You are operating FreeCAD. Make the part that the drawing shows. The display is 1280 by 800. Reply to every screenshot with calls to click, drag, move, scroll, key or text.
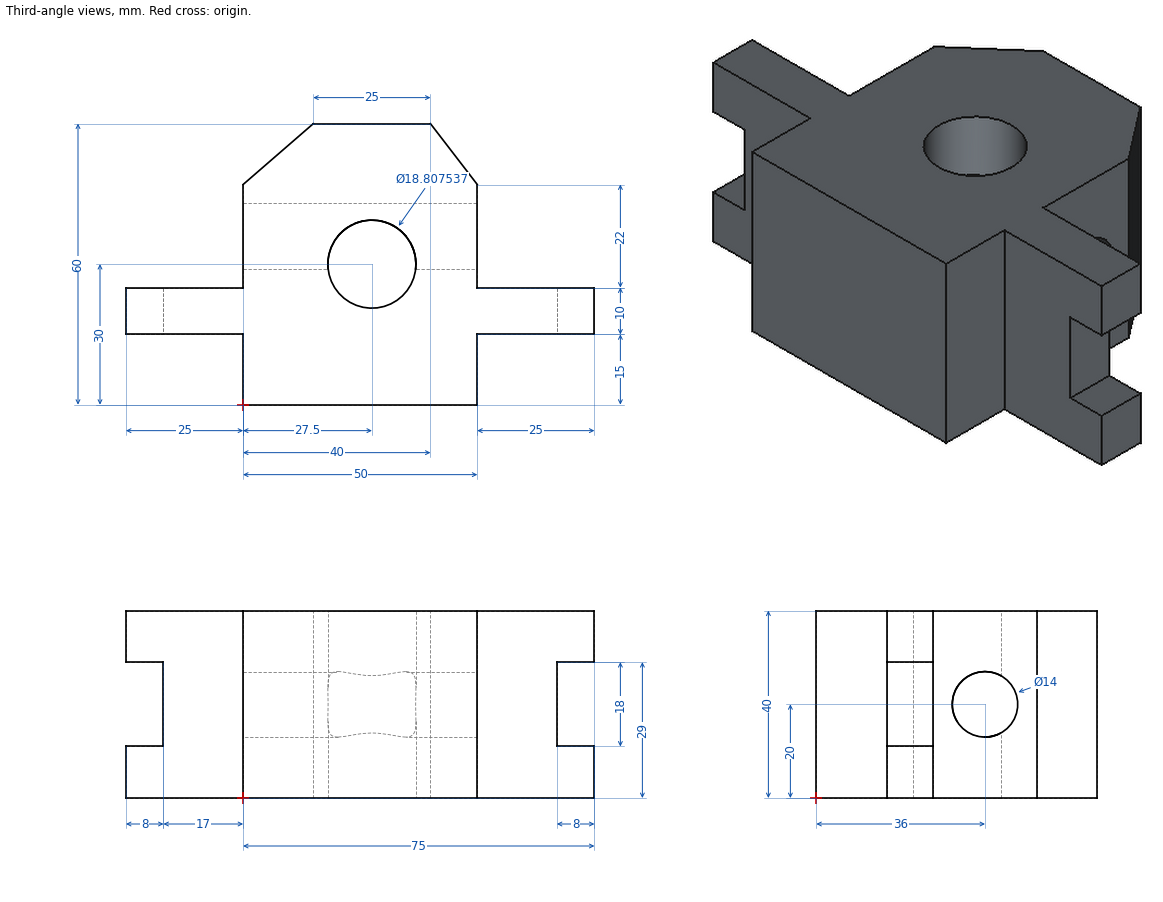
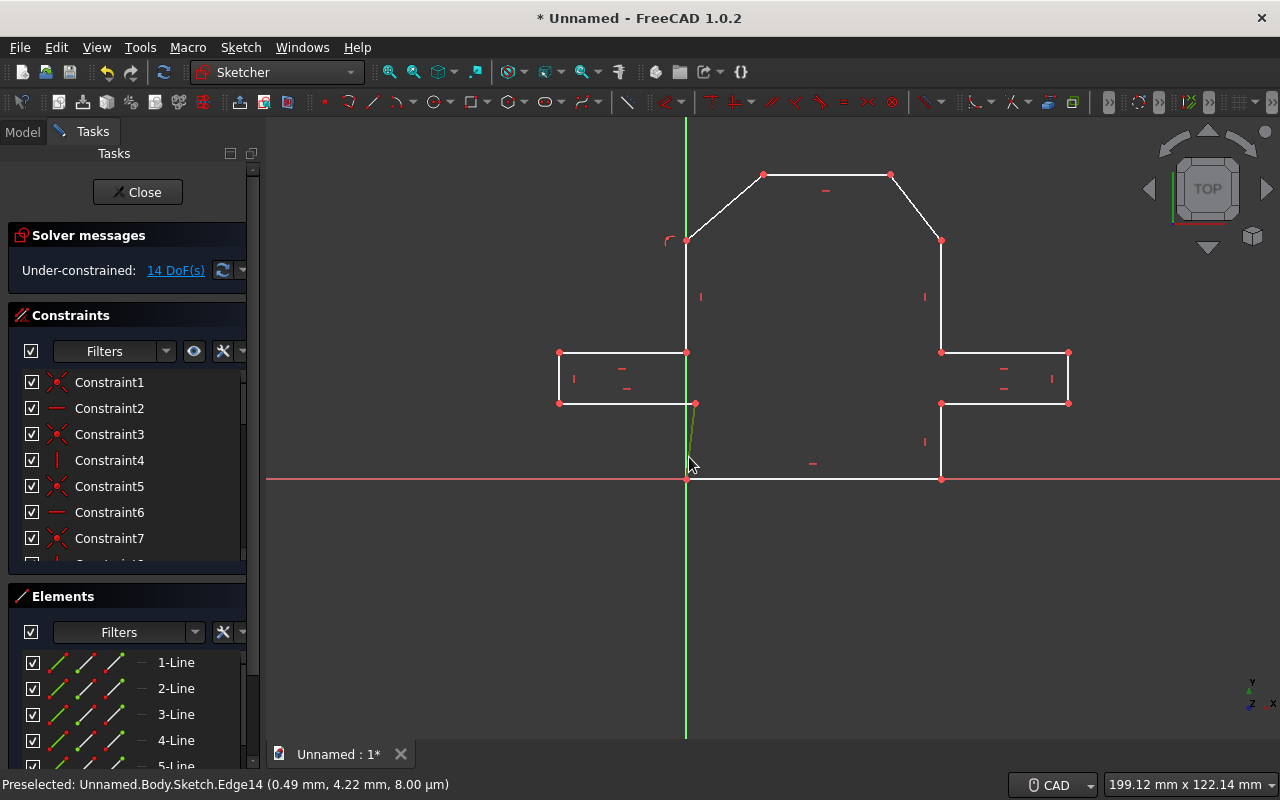
key(v)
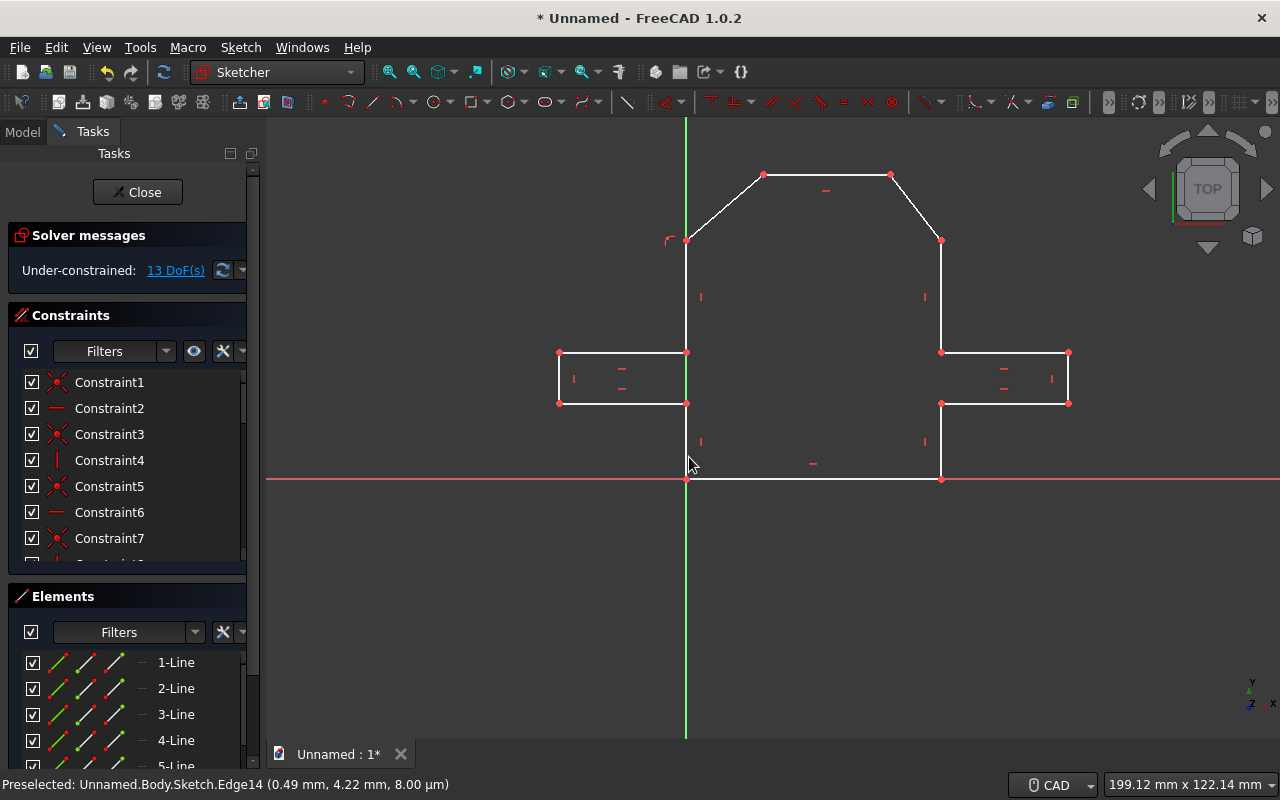
click(763, 479)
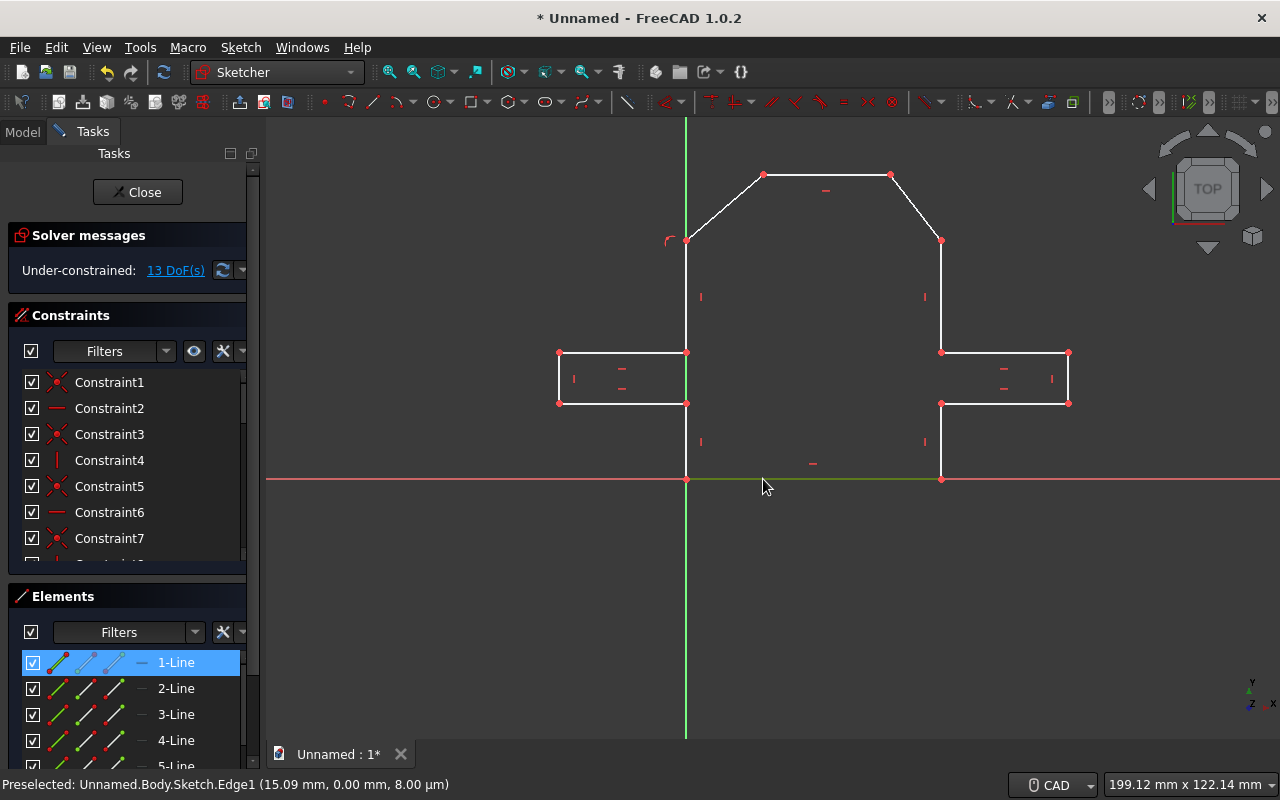
click(684, 102)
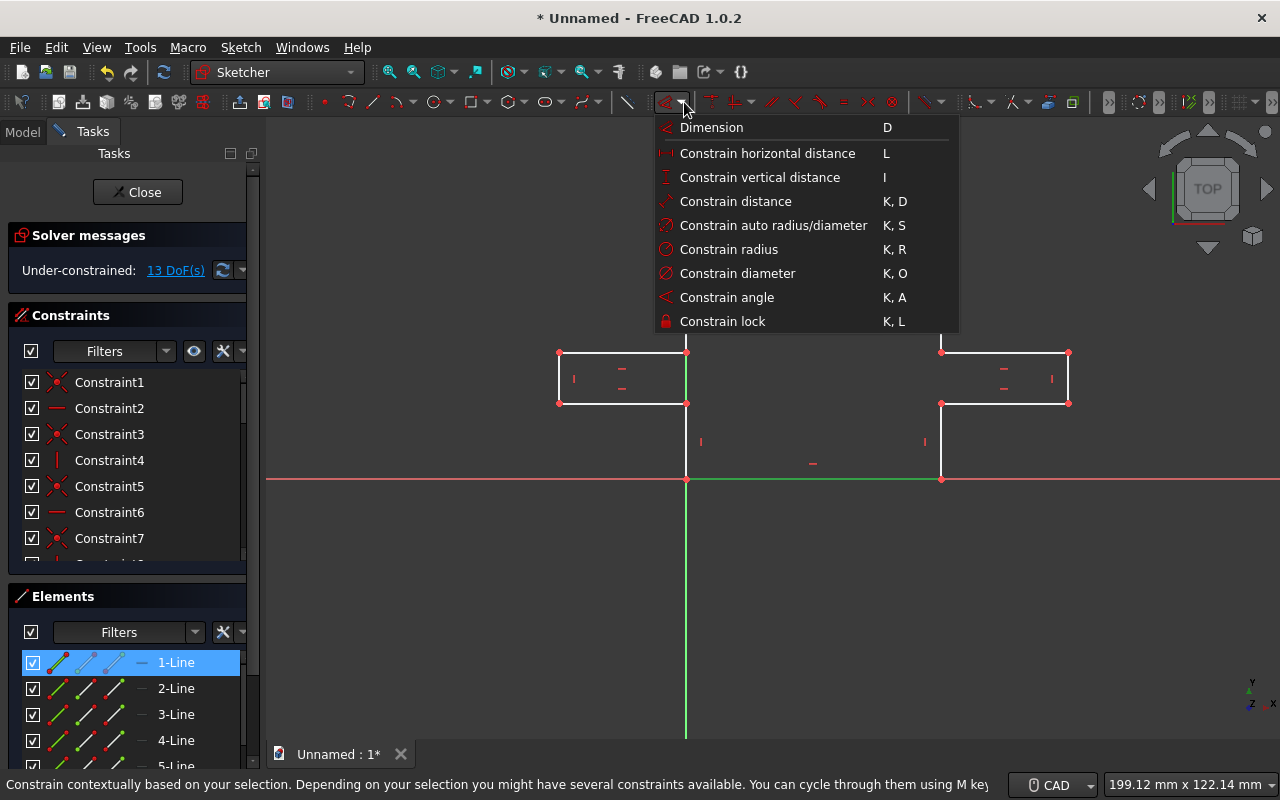
click(807, 153)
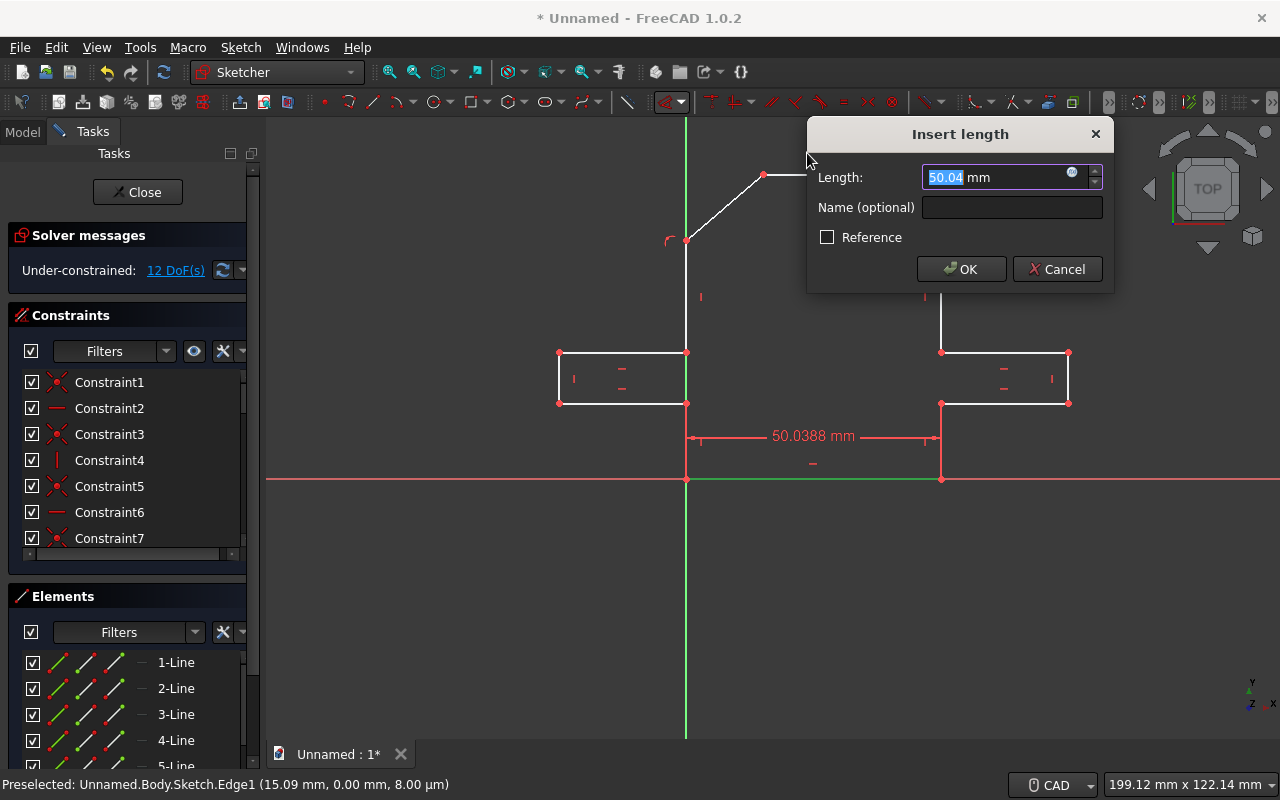
text(50)
key(Return)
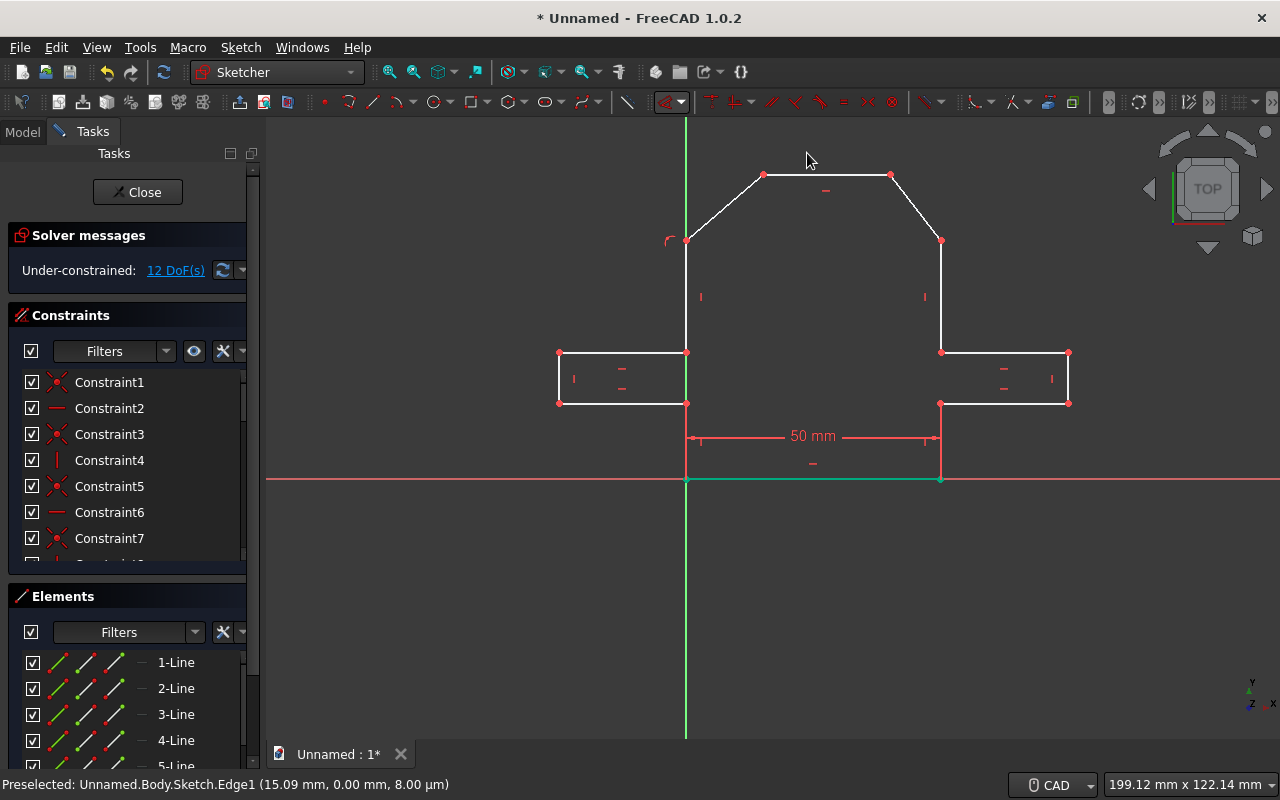
click(941, 457)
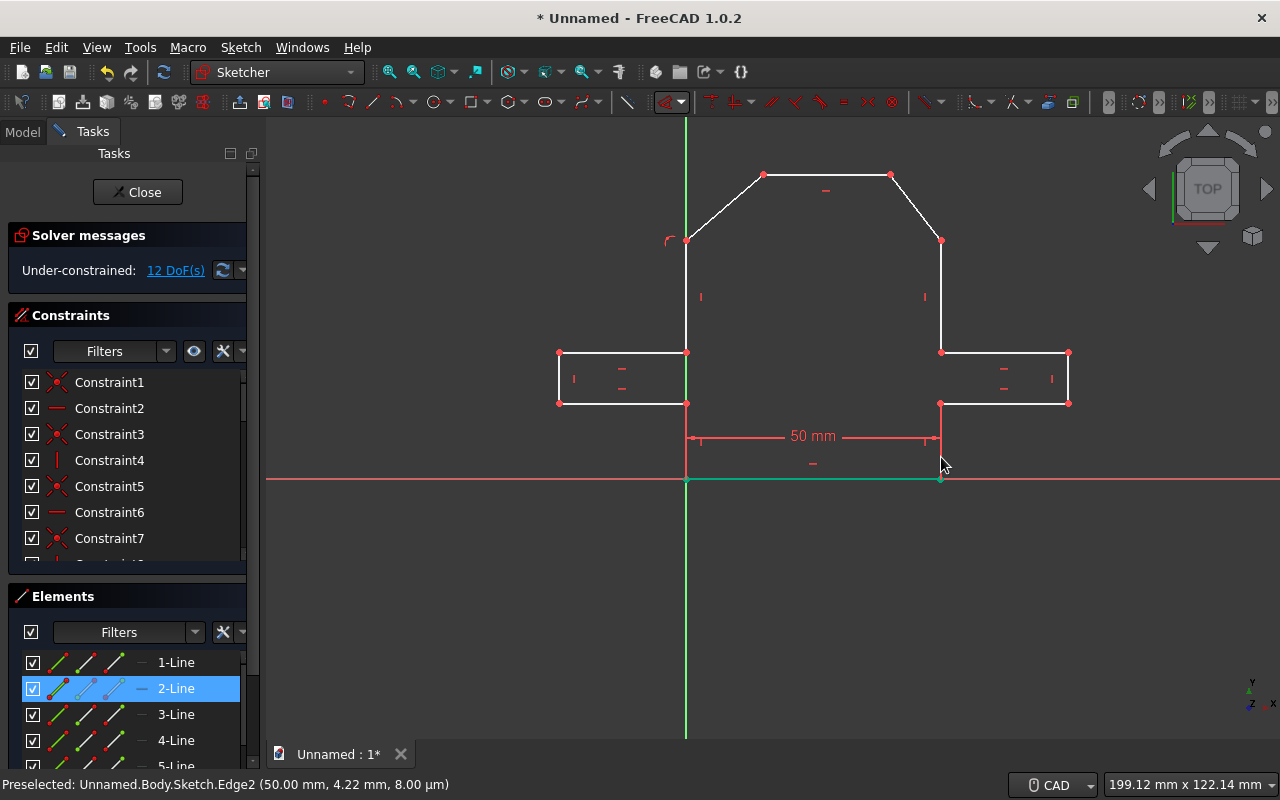
key(i)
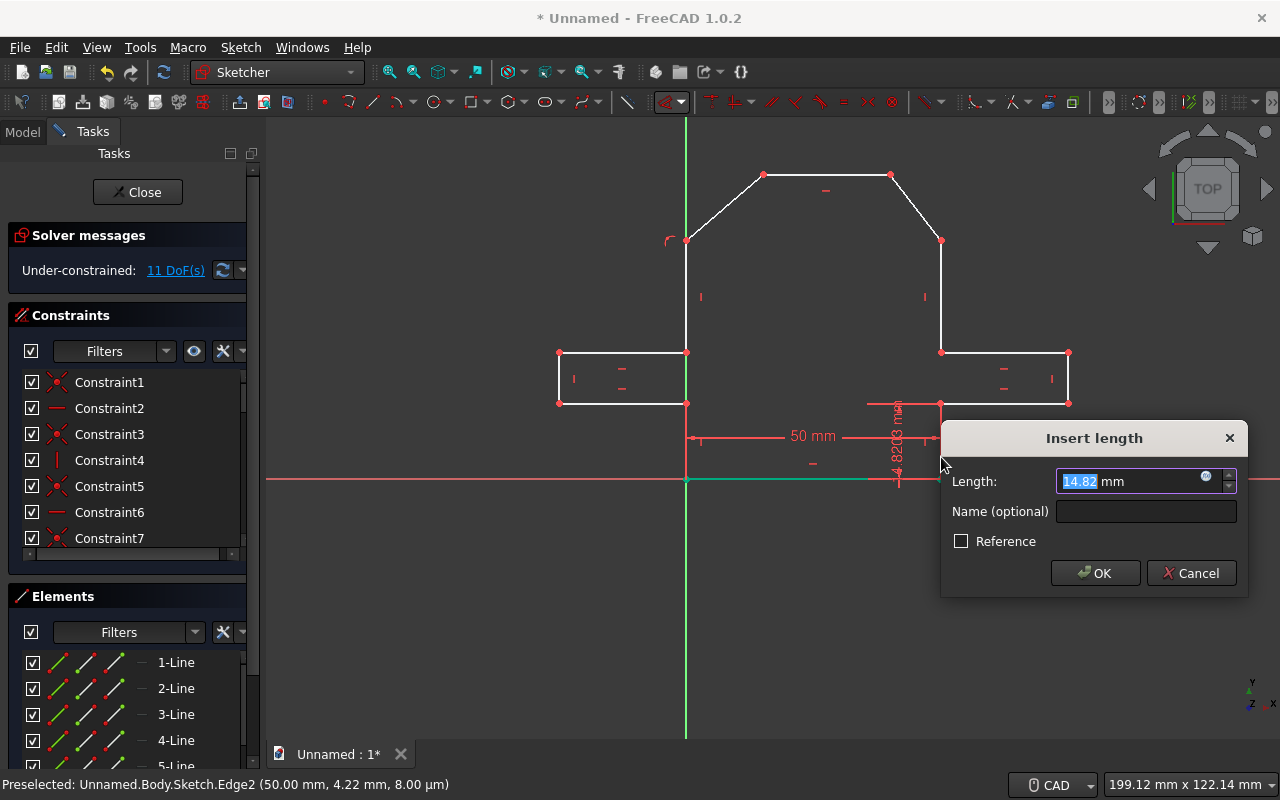
text(15)
key(Return)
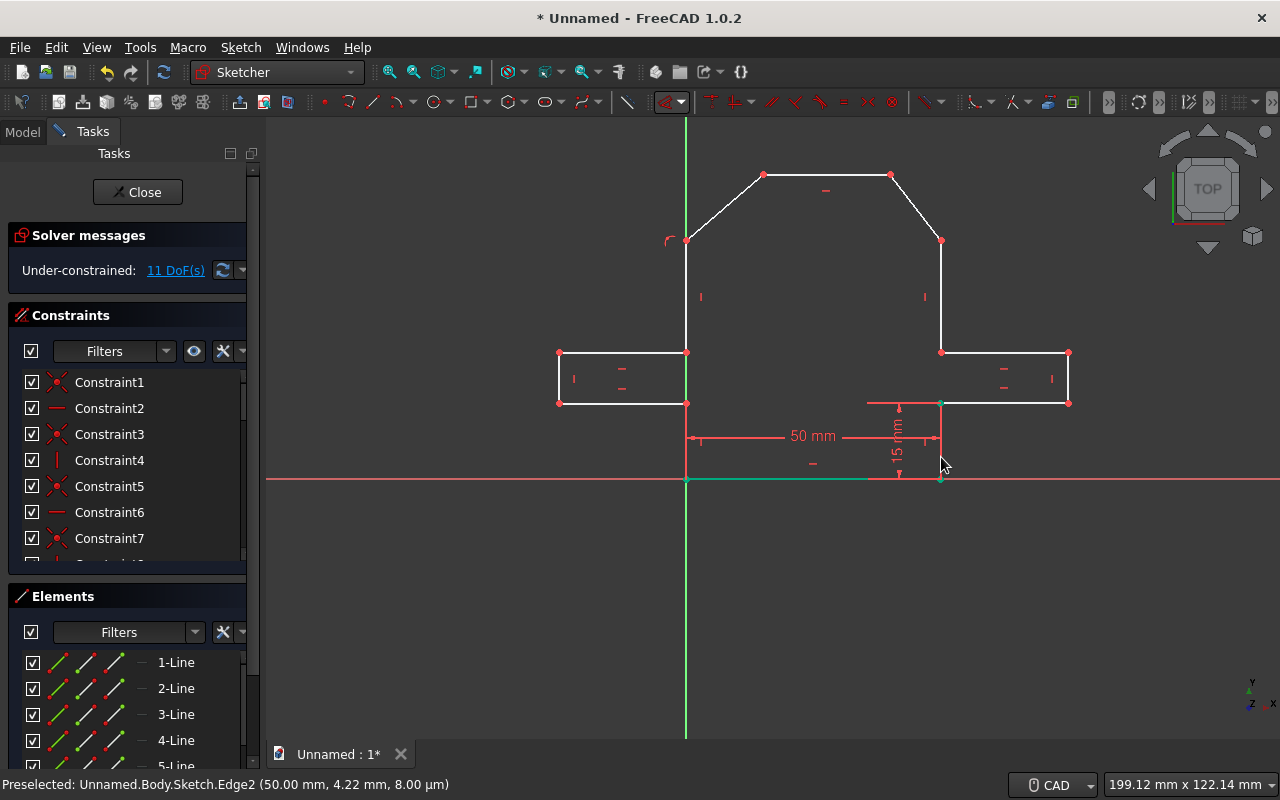
click(979, 403)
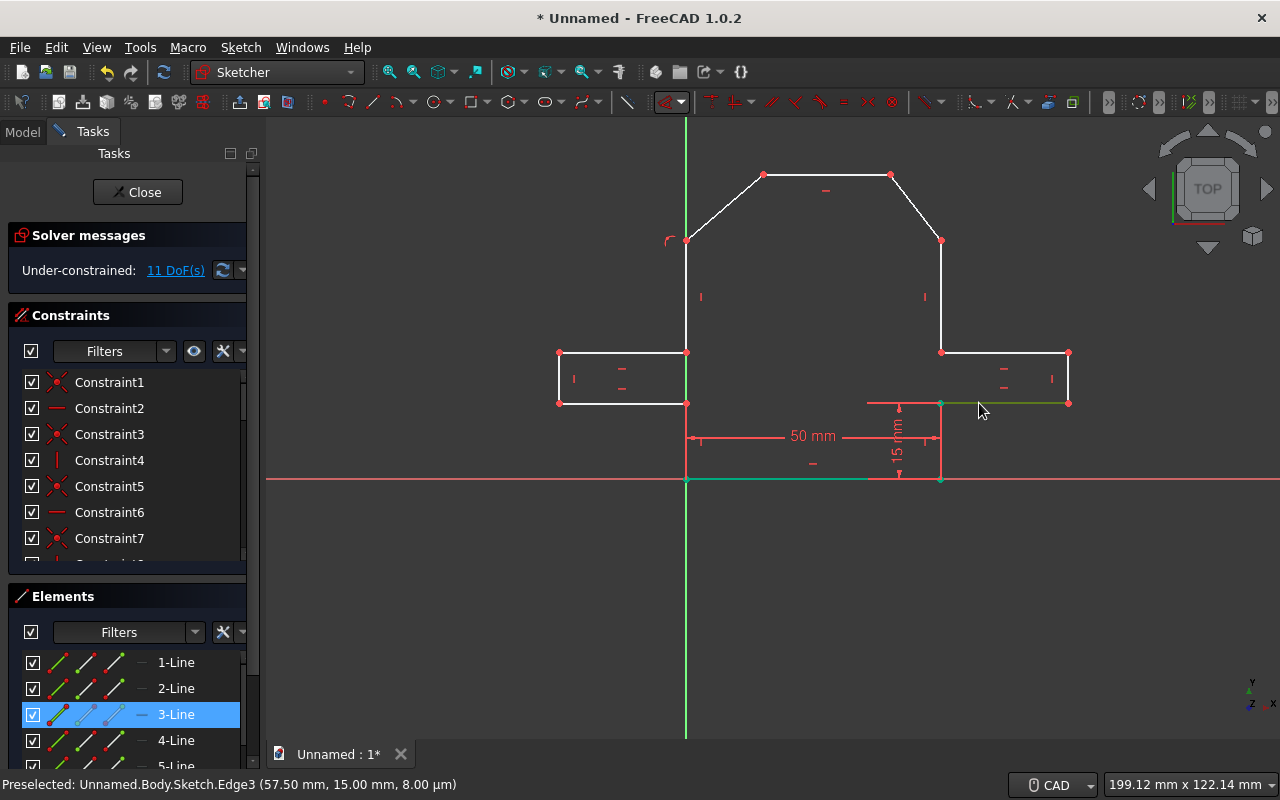
key(l)